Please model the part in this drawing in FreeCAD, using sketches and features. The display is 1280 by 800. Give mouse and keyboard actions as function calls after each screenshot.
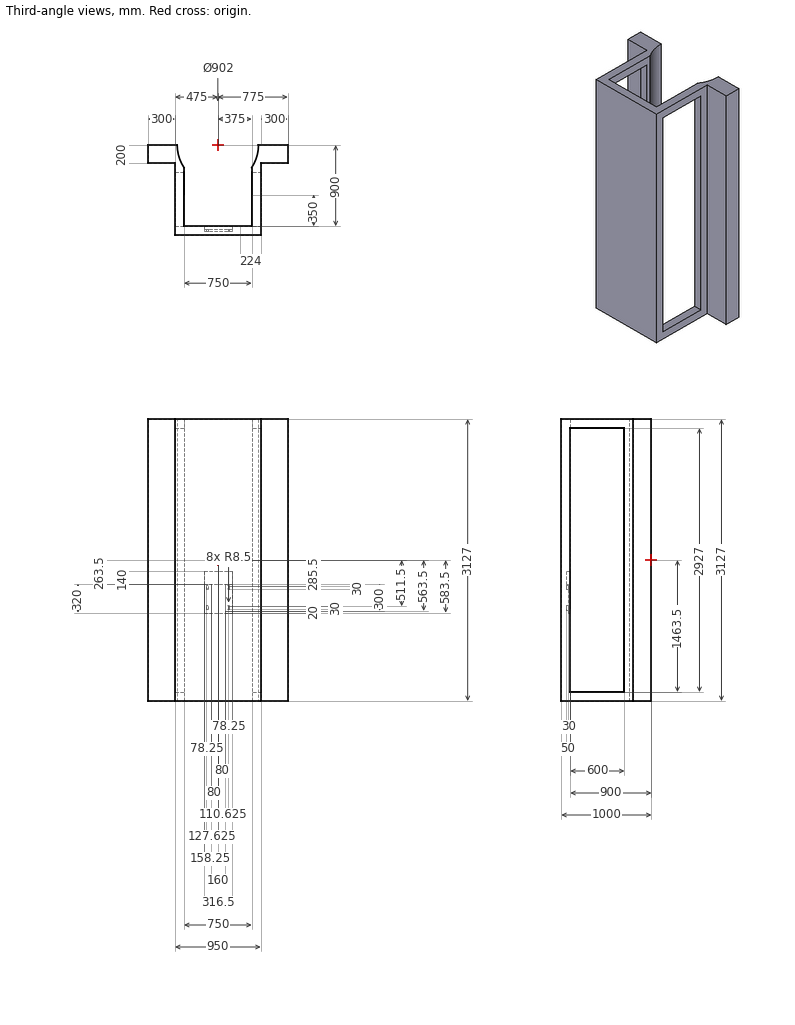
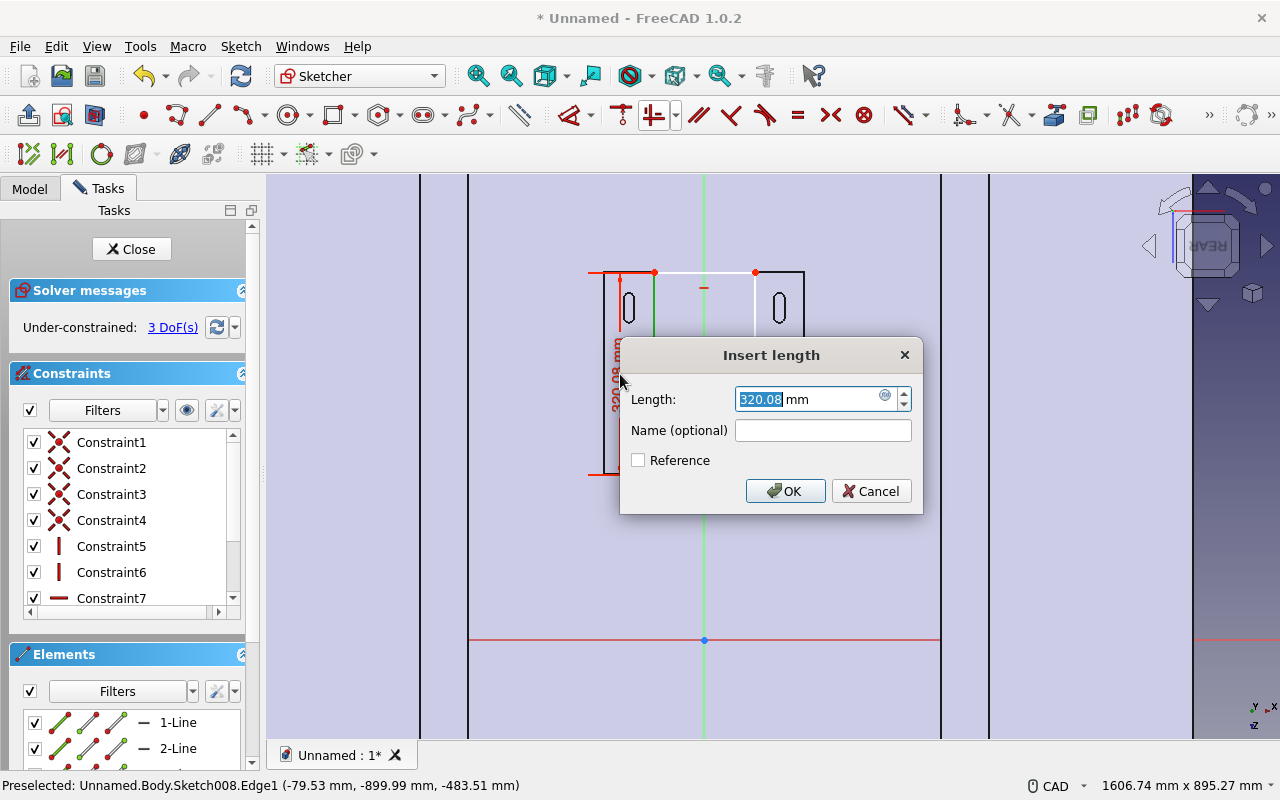
text(320)
key(Return)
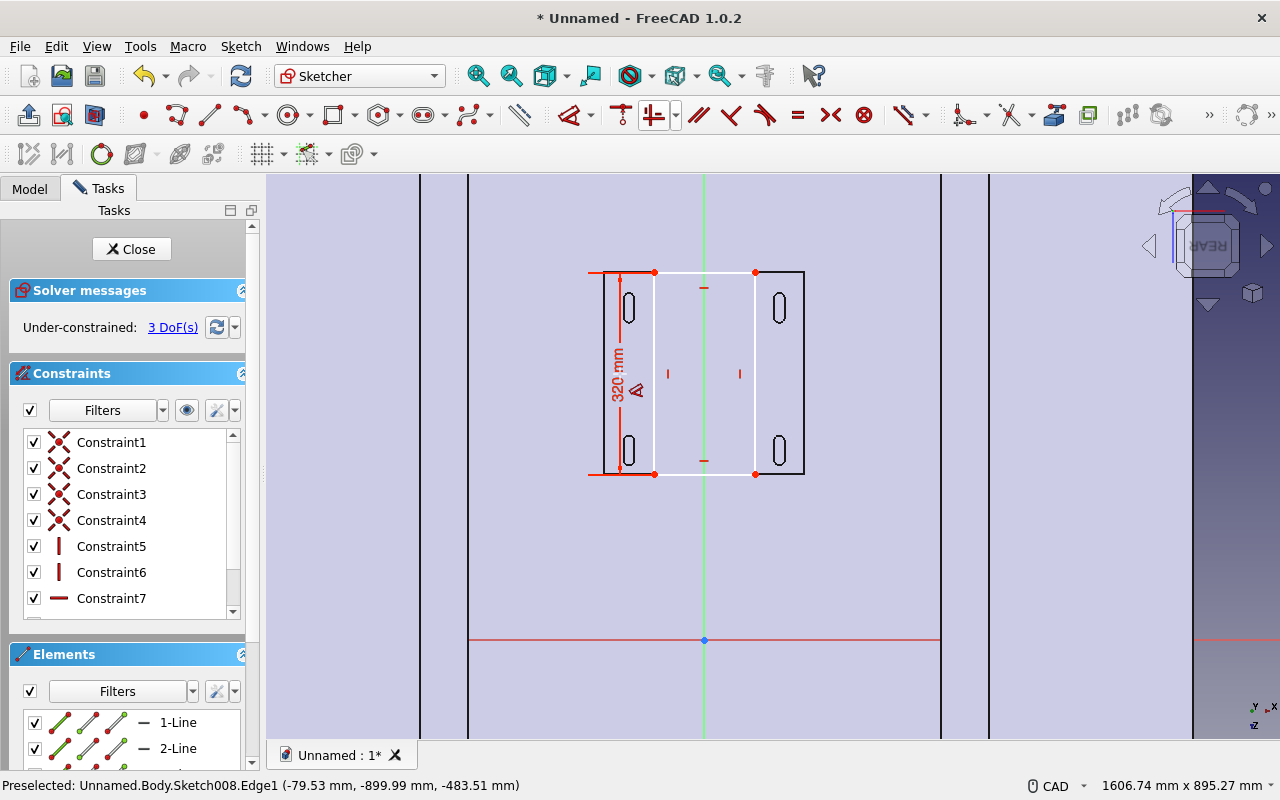
click(684, 475)
click(681, 509)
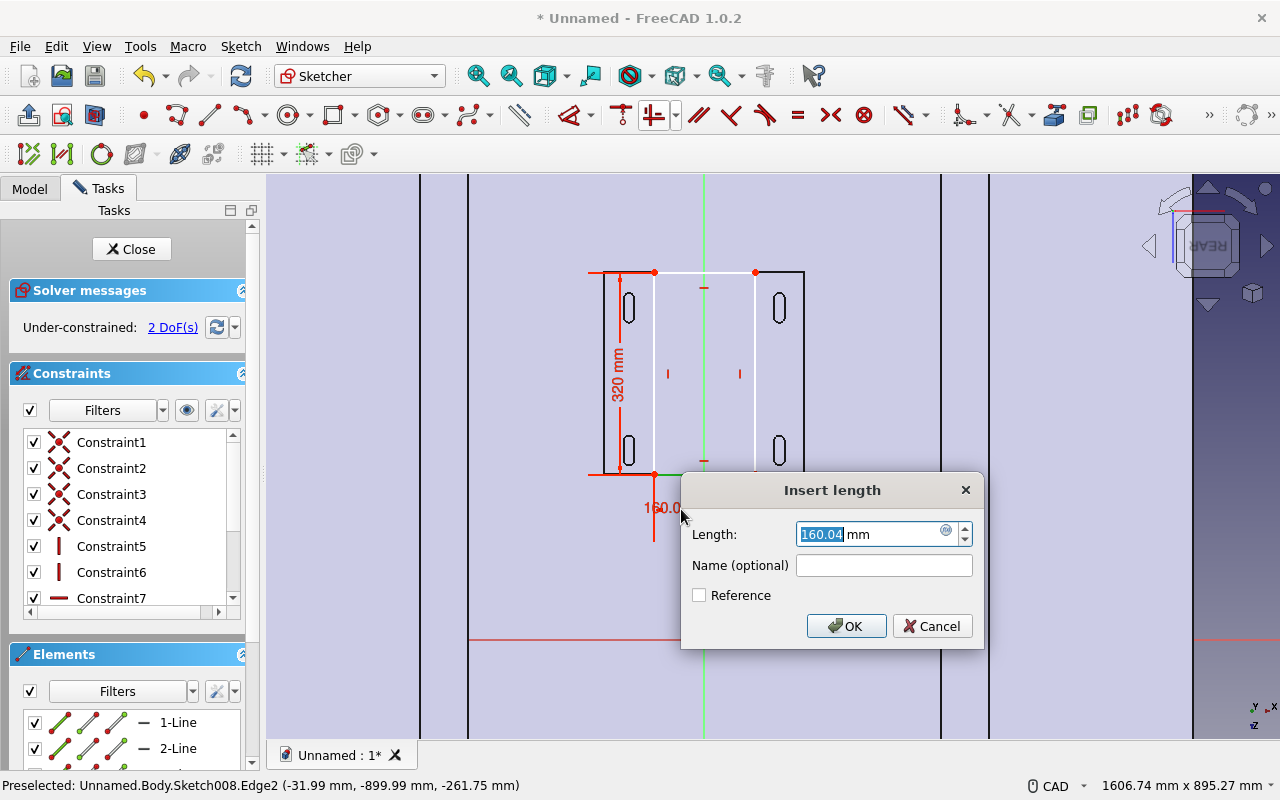
text(160)
key(Return)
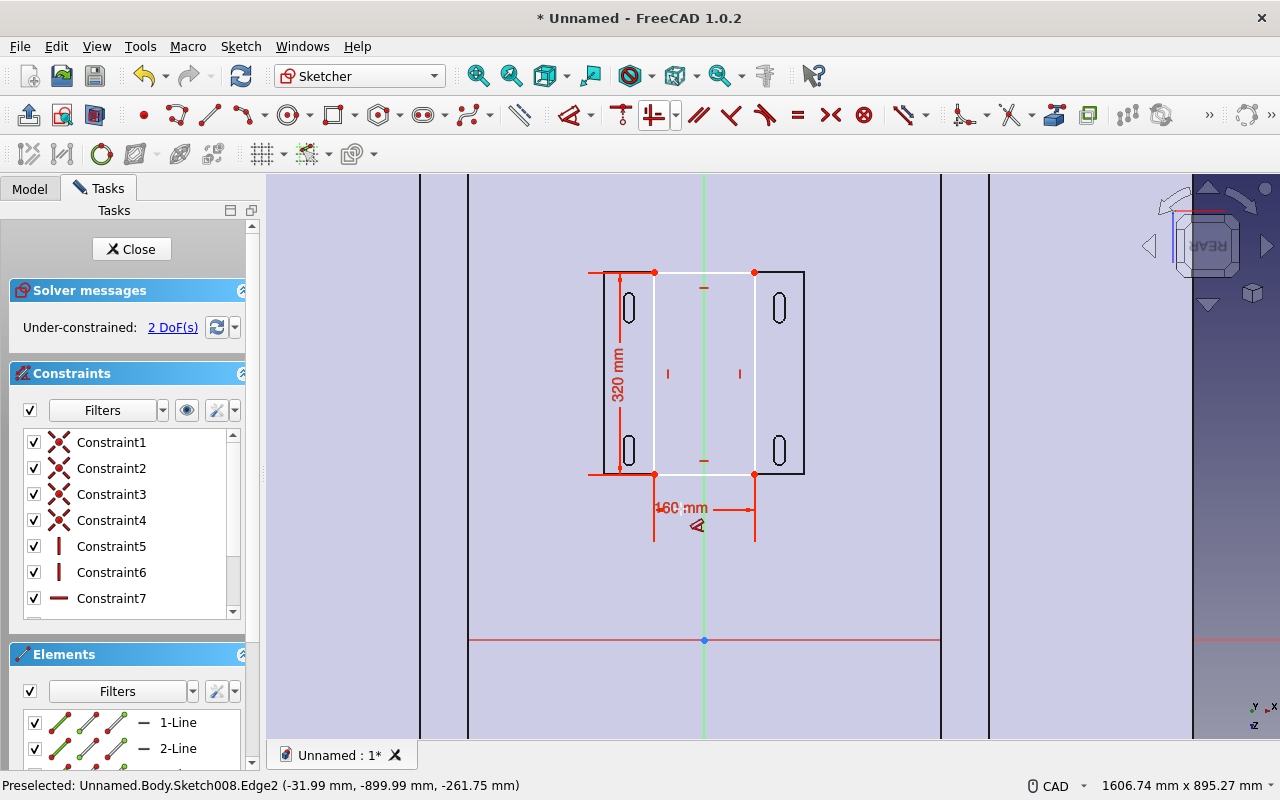
click(654, 273)
click(679, 674)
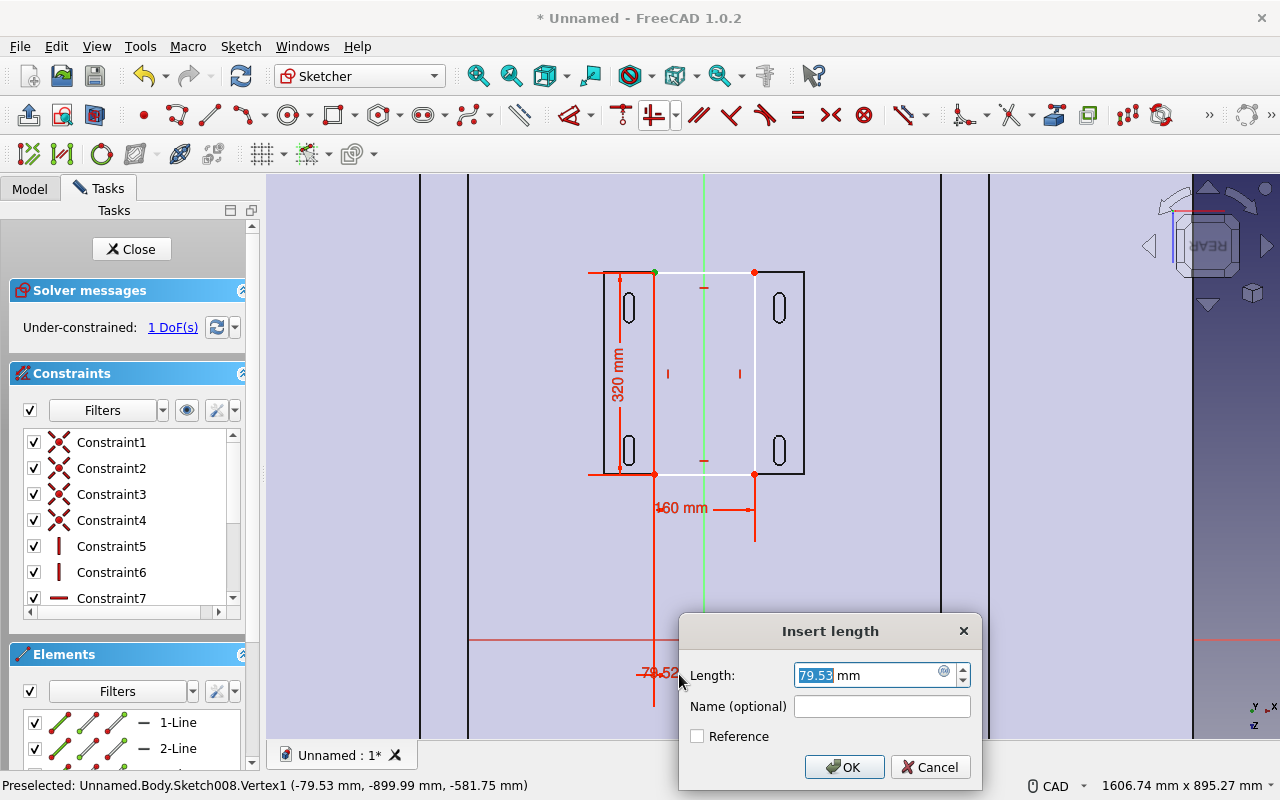
text(80)
key(Return)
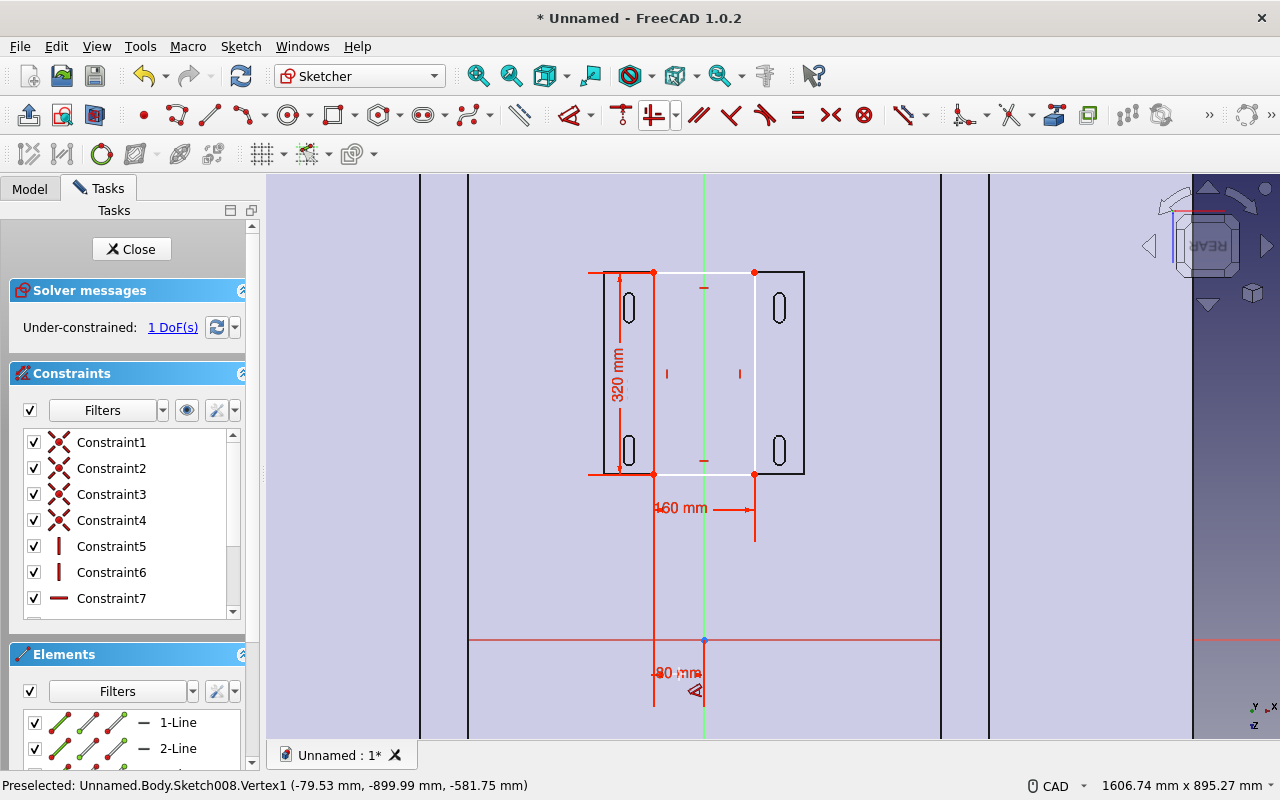
click(654, 273)
click(620, 457)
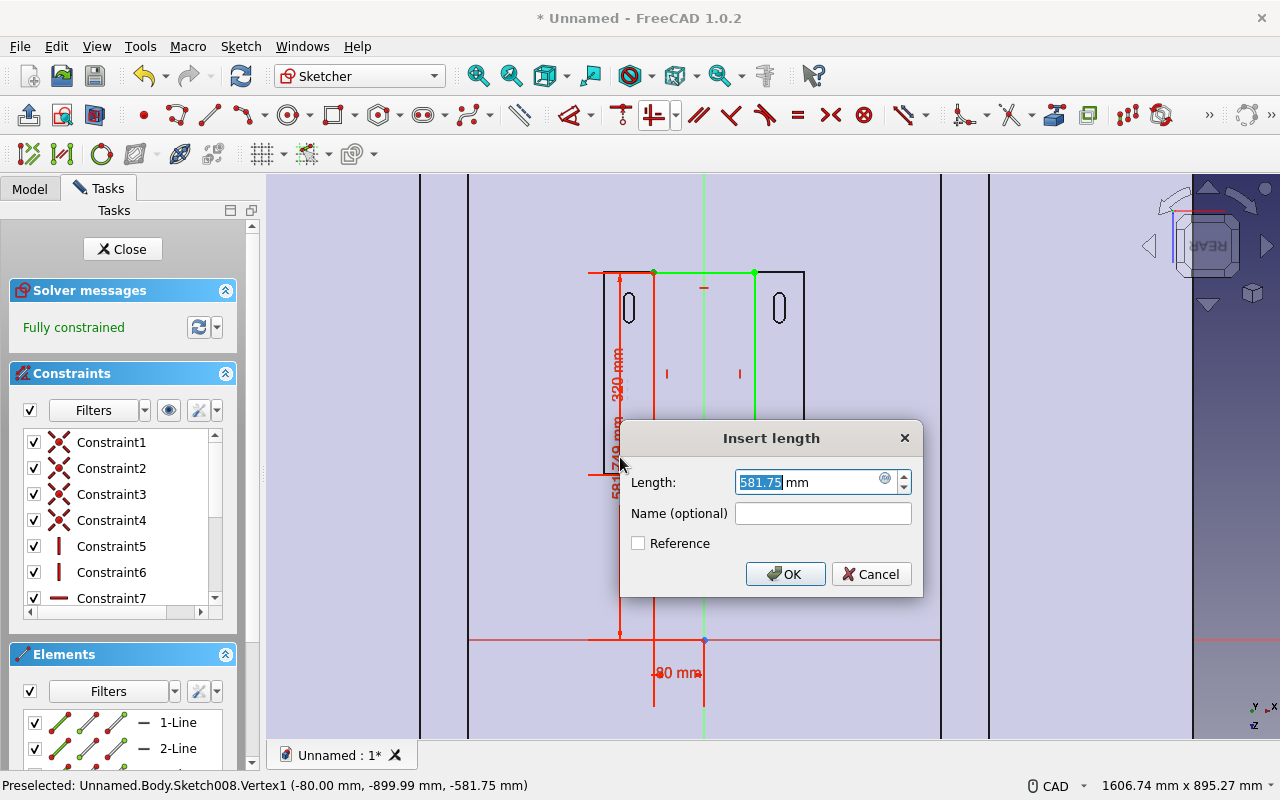
text(583.5)
key(Return)
key(Escape)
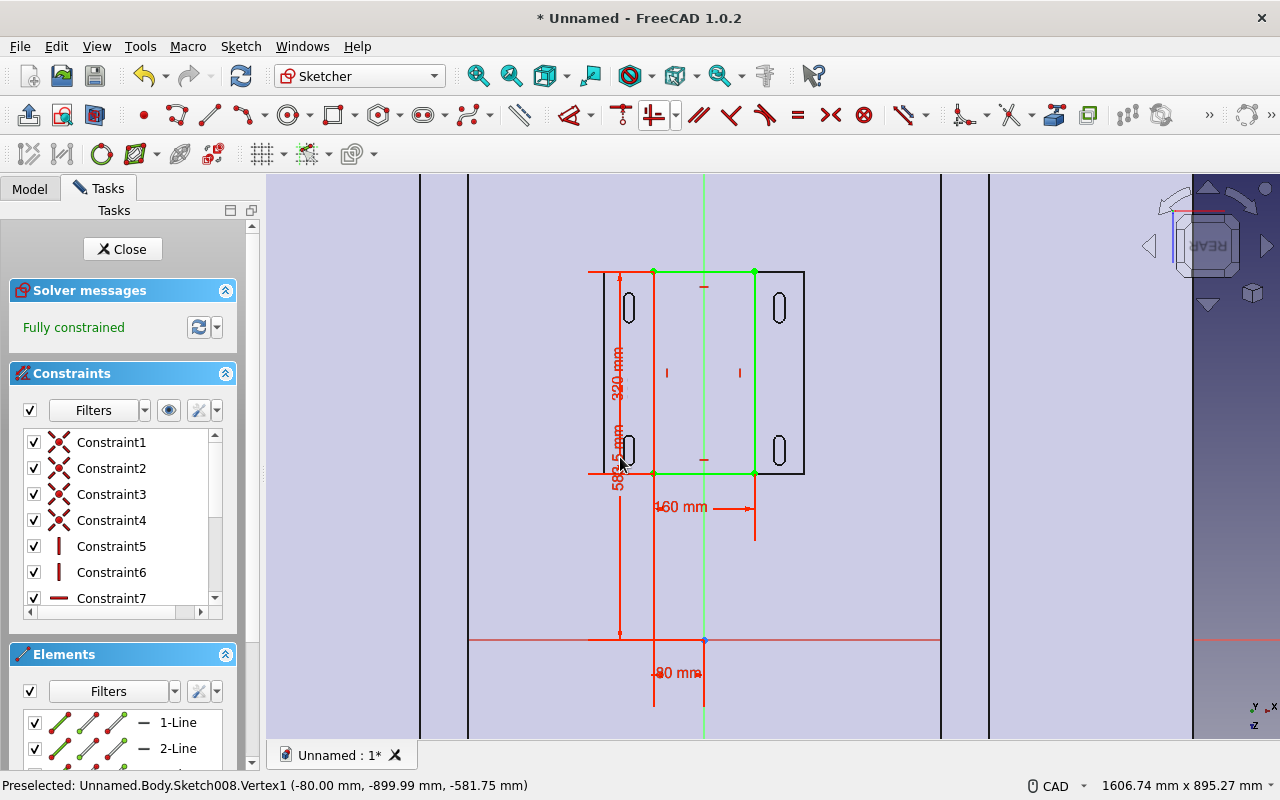
click(123, 249)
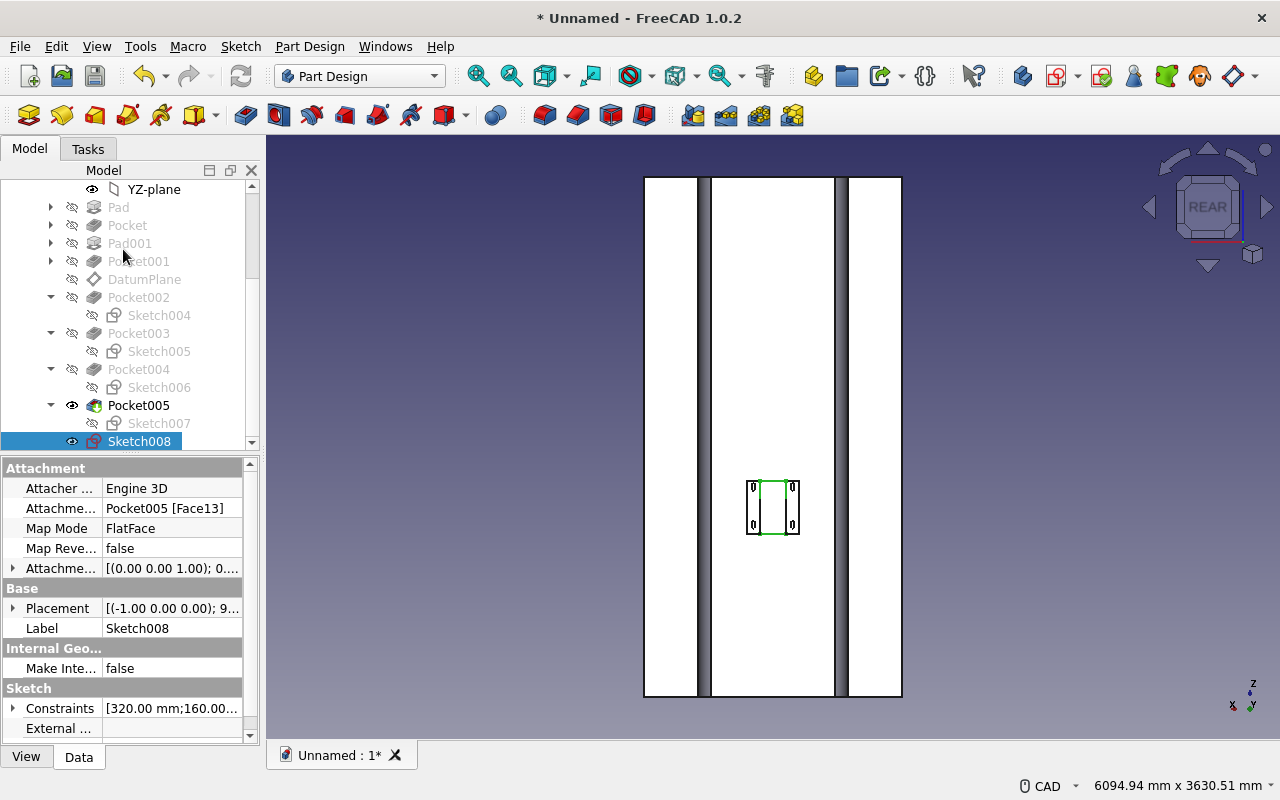
click(246, 116)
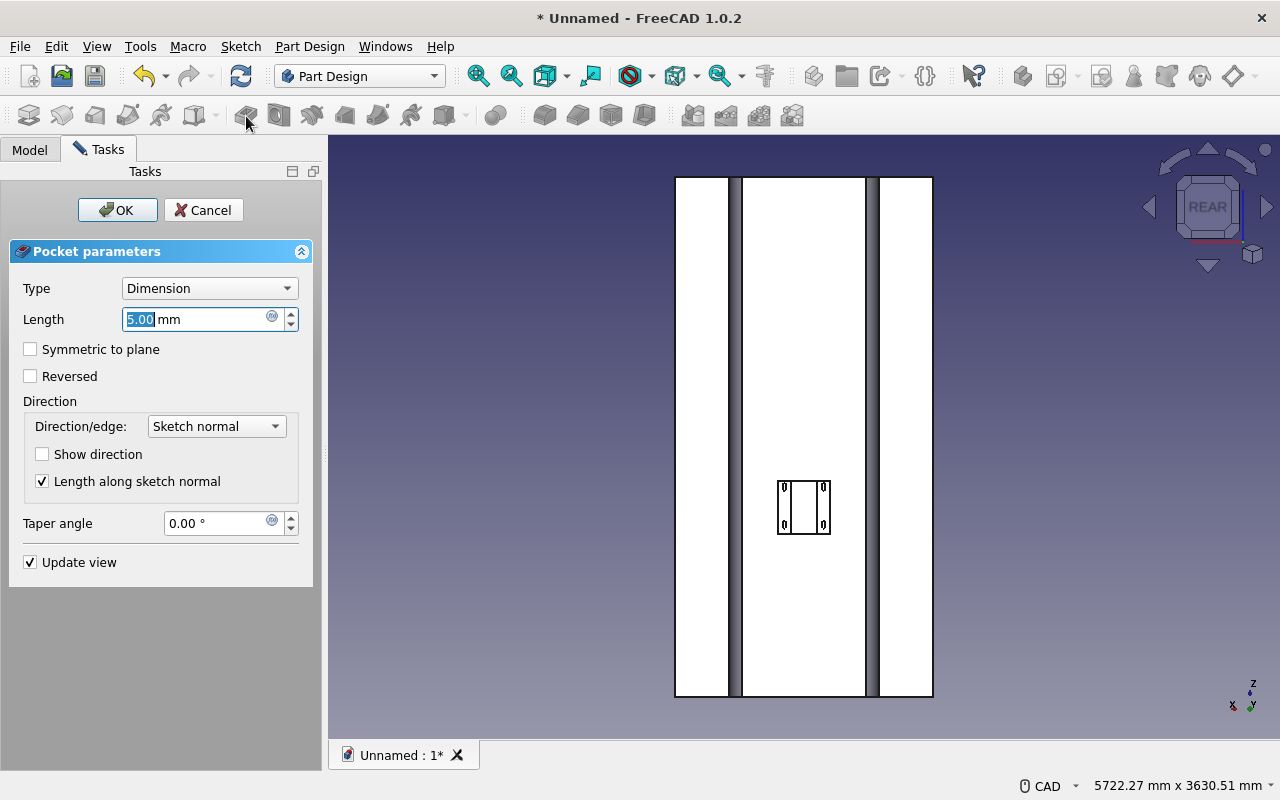
text(30)
key(Tab)